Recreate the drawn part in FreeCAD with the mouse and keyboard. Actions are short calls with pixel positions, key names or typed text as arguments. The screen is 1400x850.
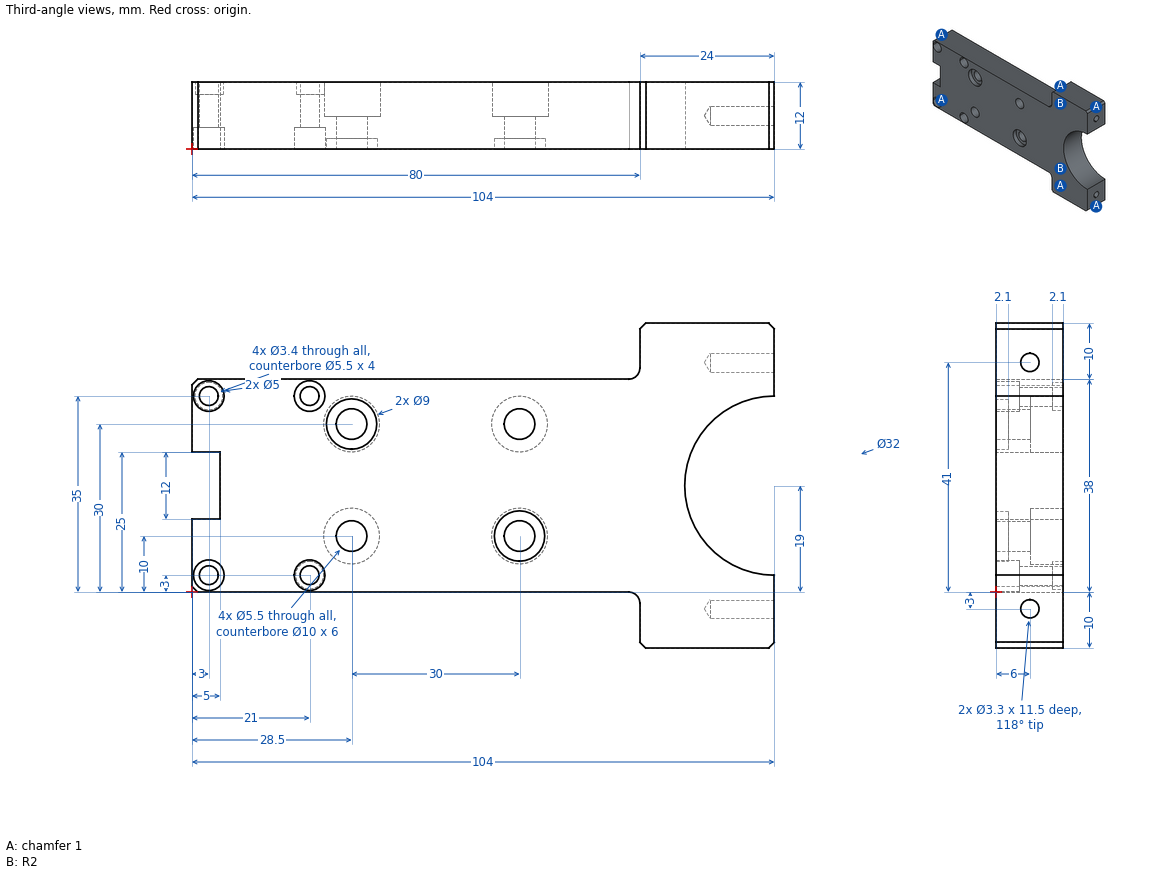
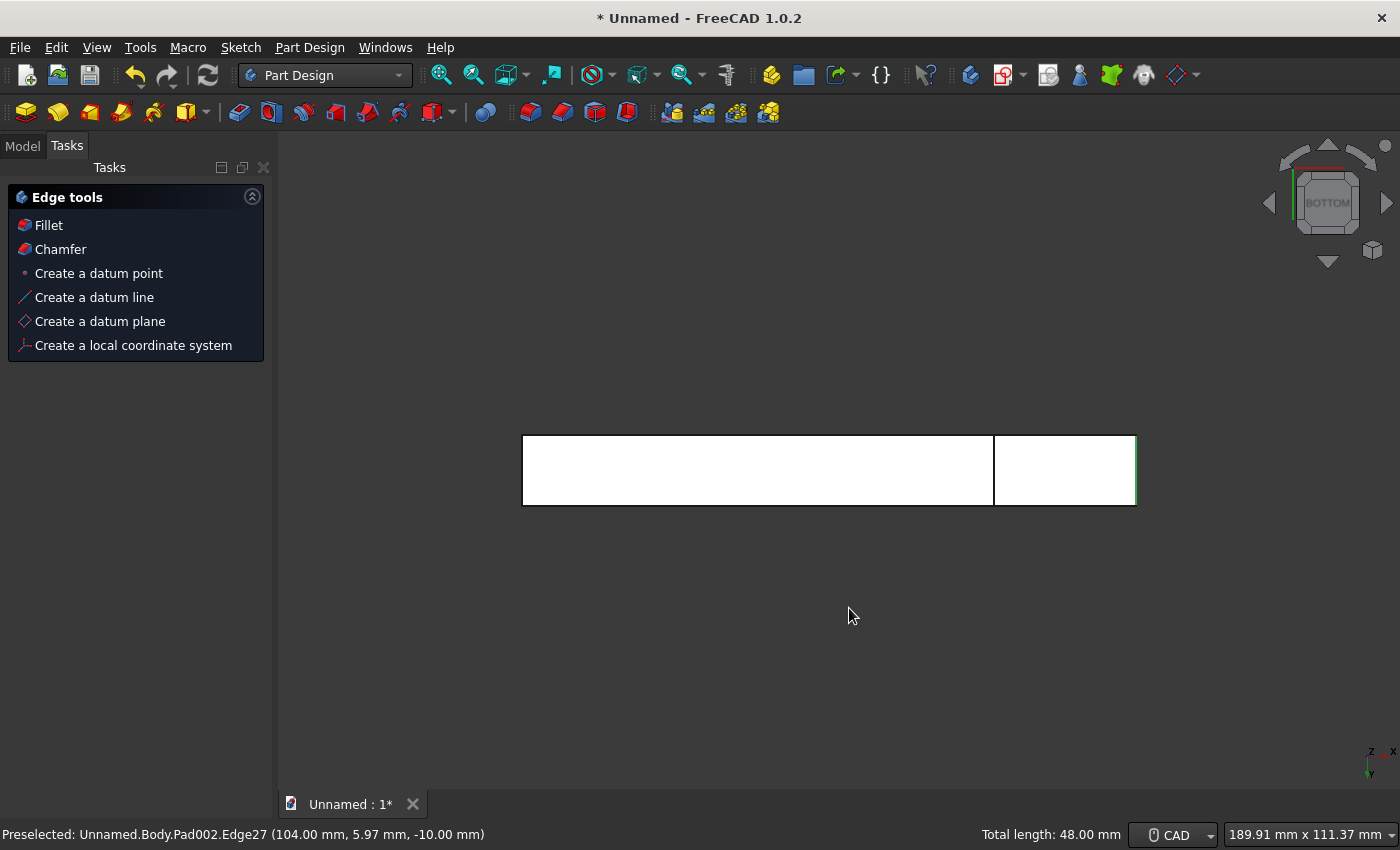
click(522, 469, ctrl)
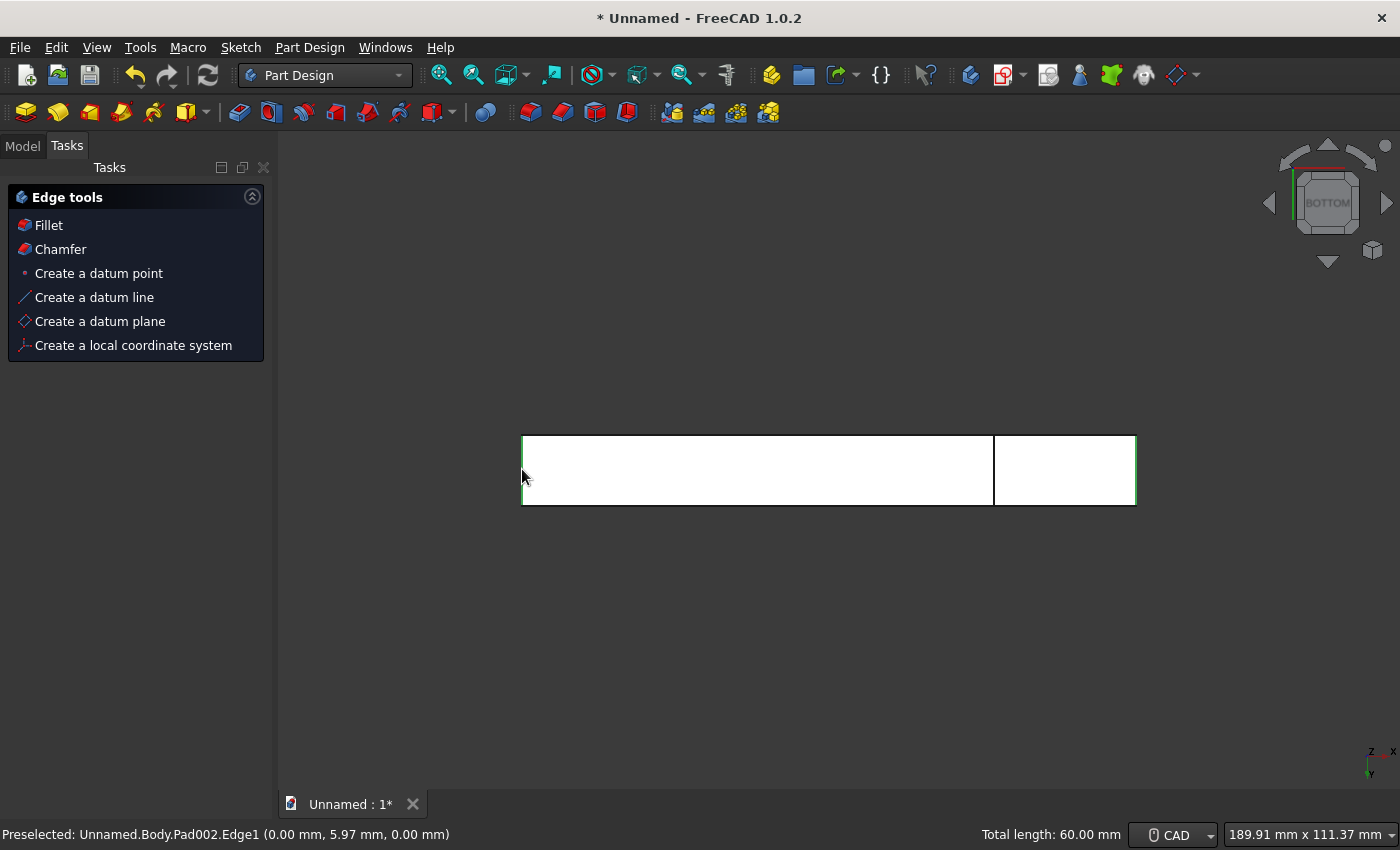
click(994, 469, ctrl)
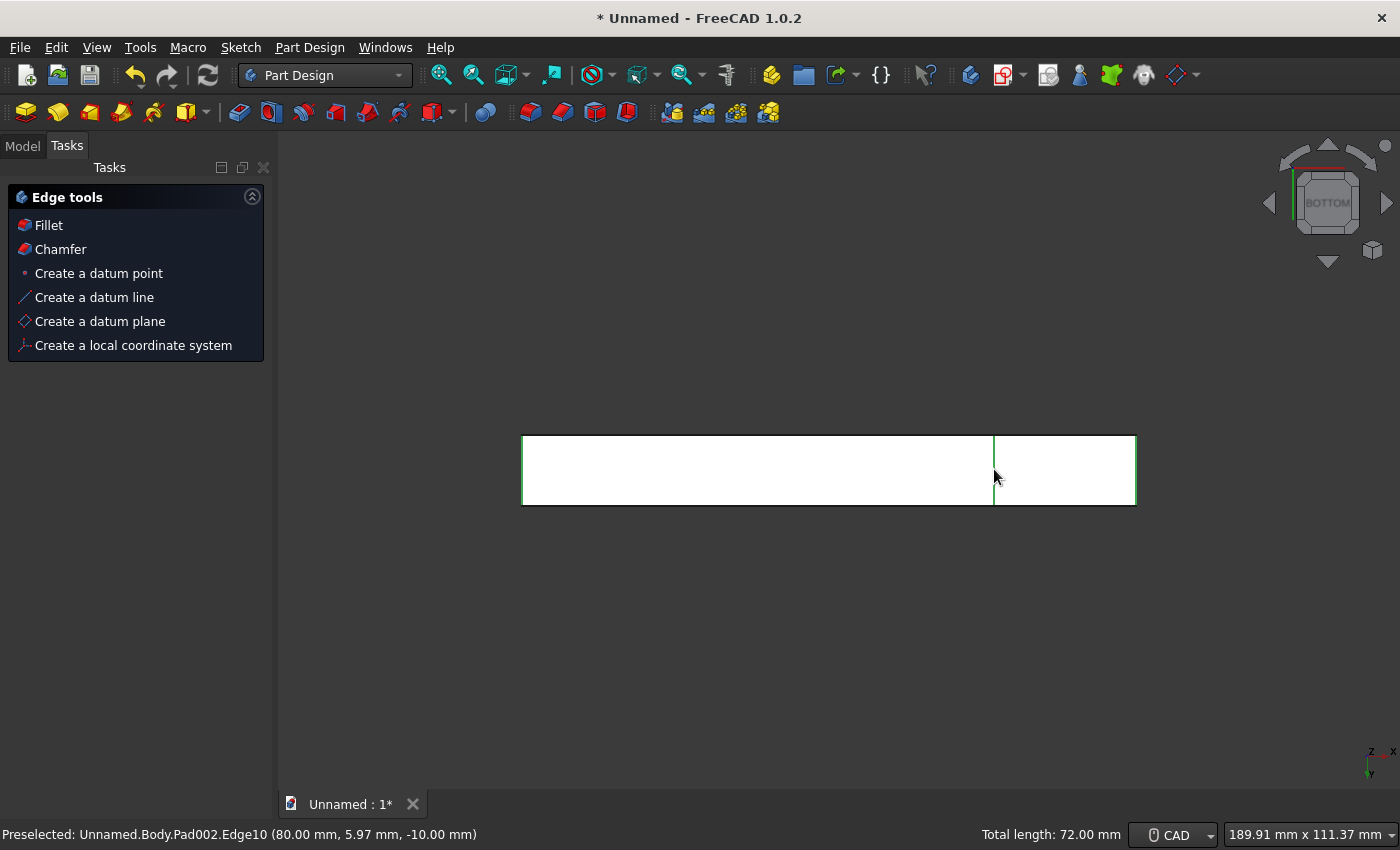
click(564, 112)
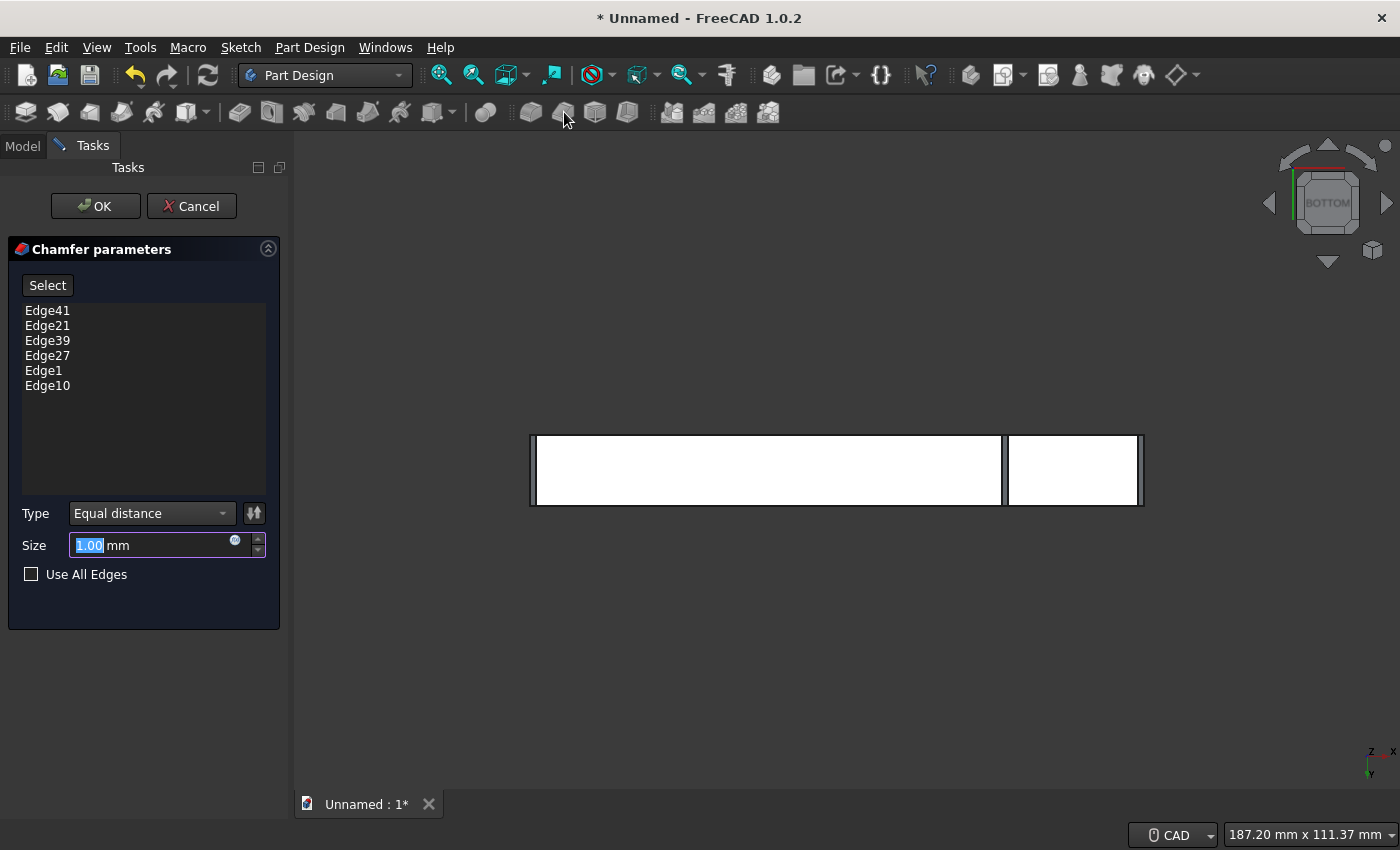
text(1)
key(Tab)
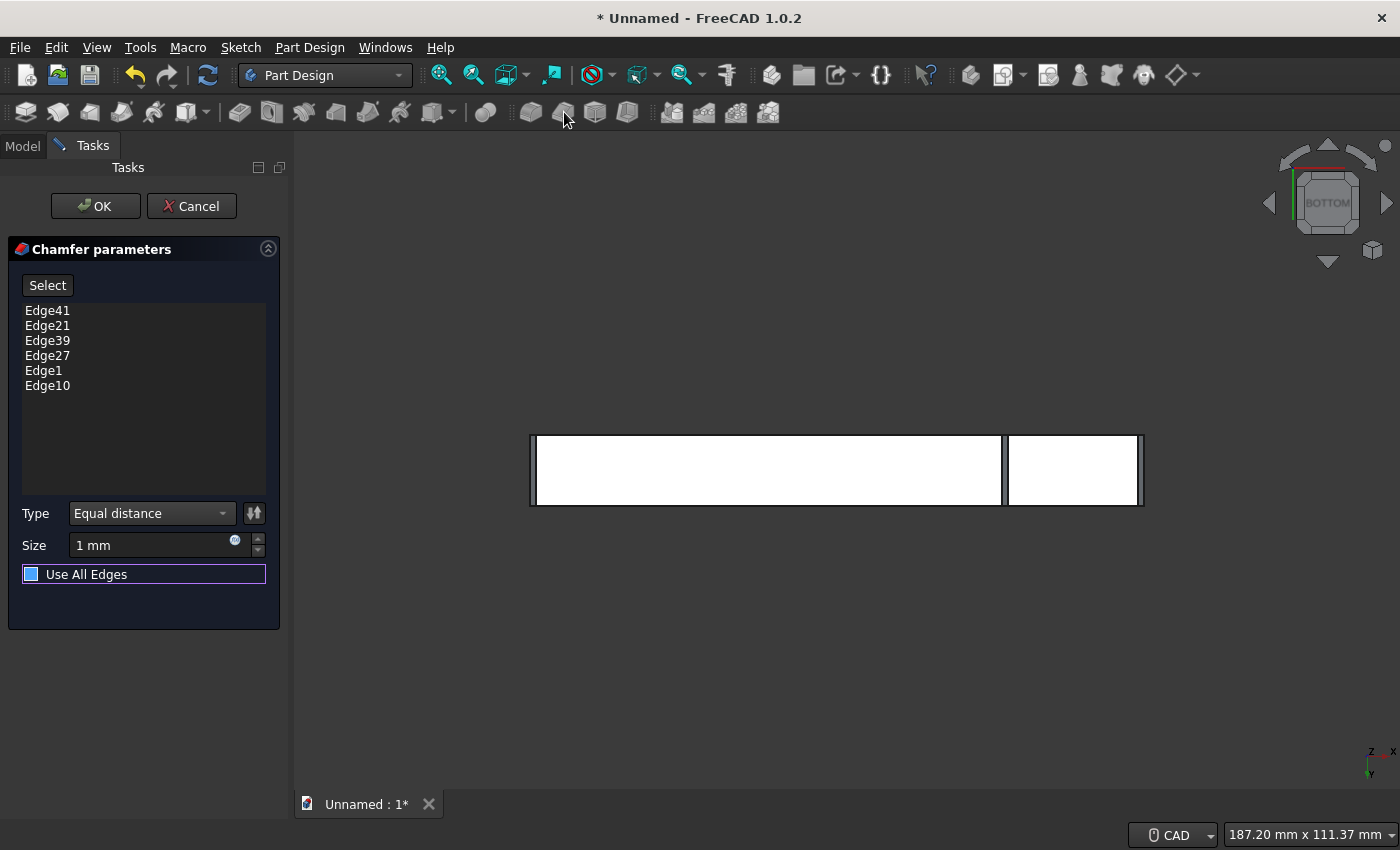
click(96, 206)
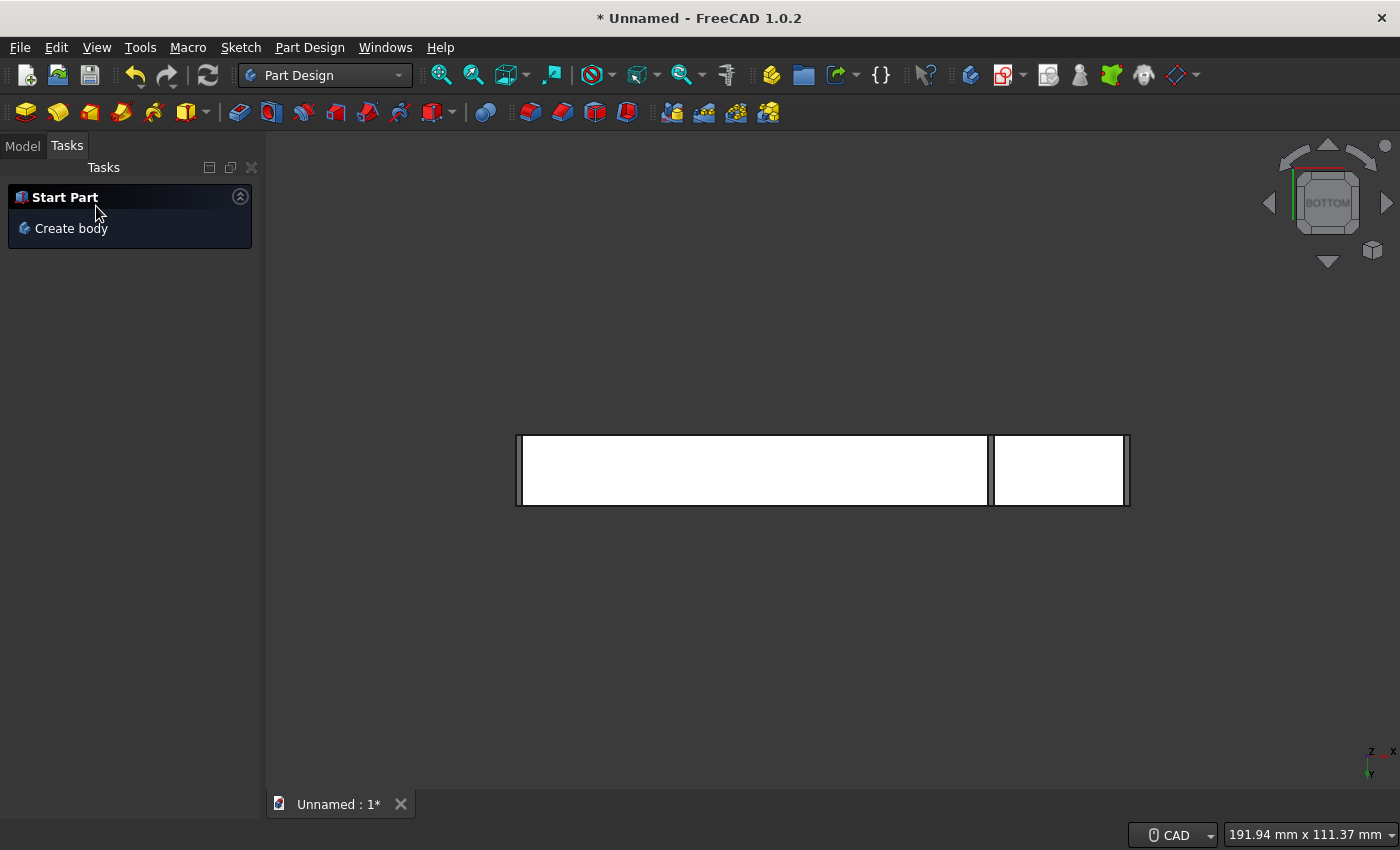
key(0)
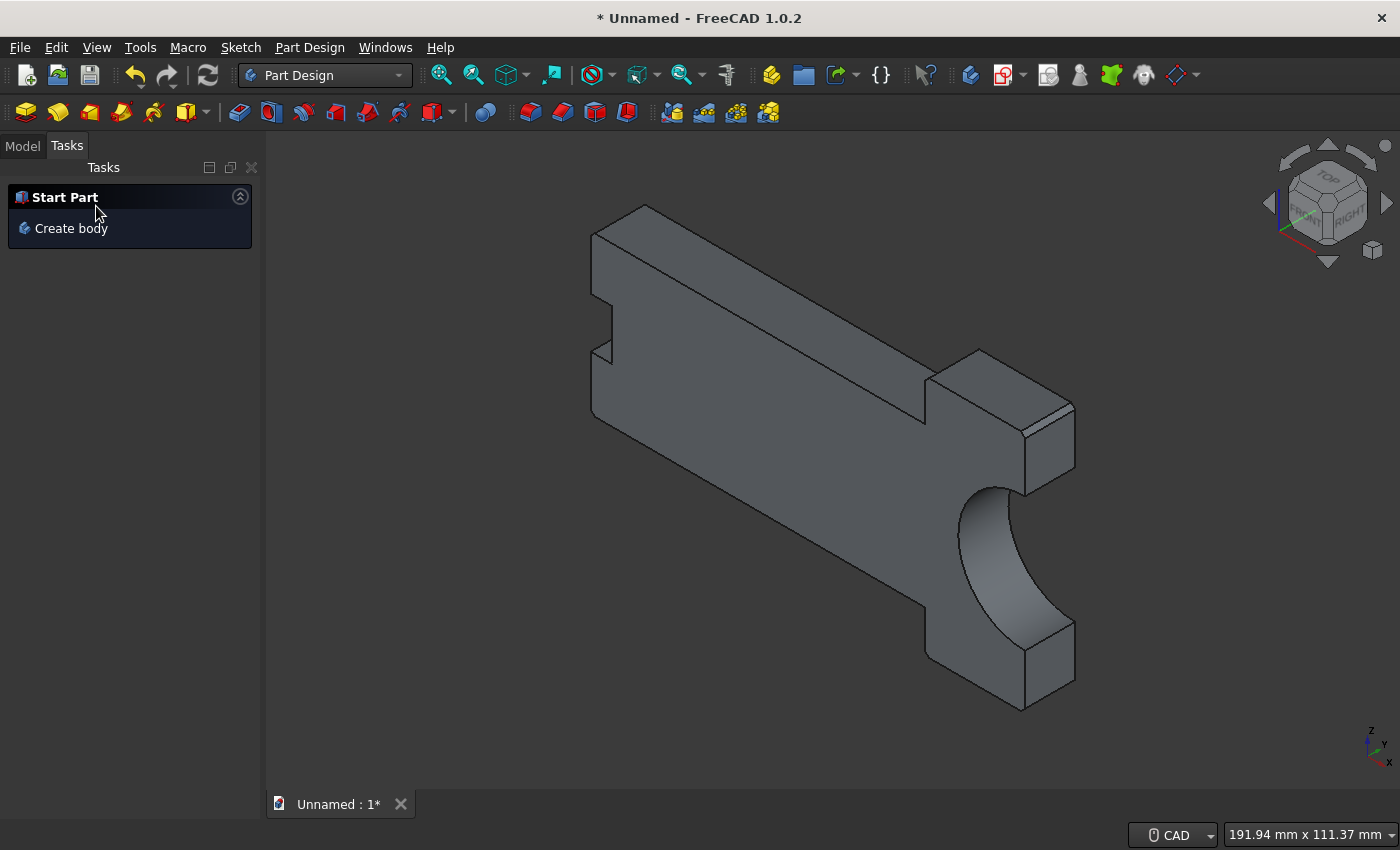
key(2)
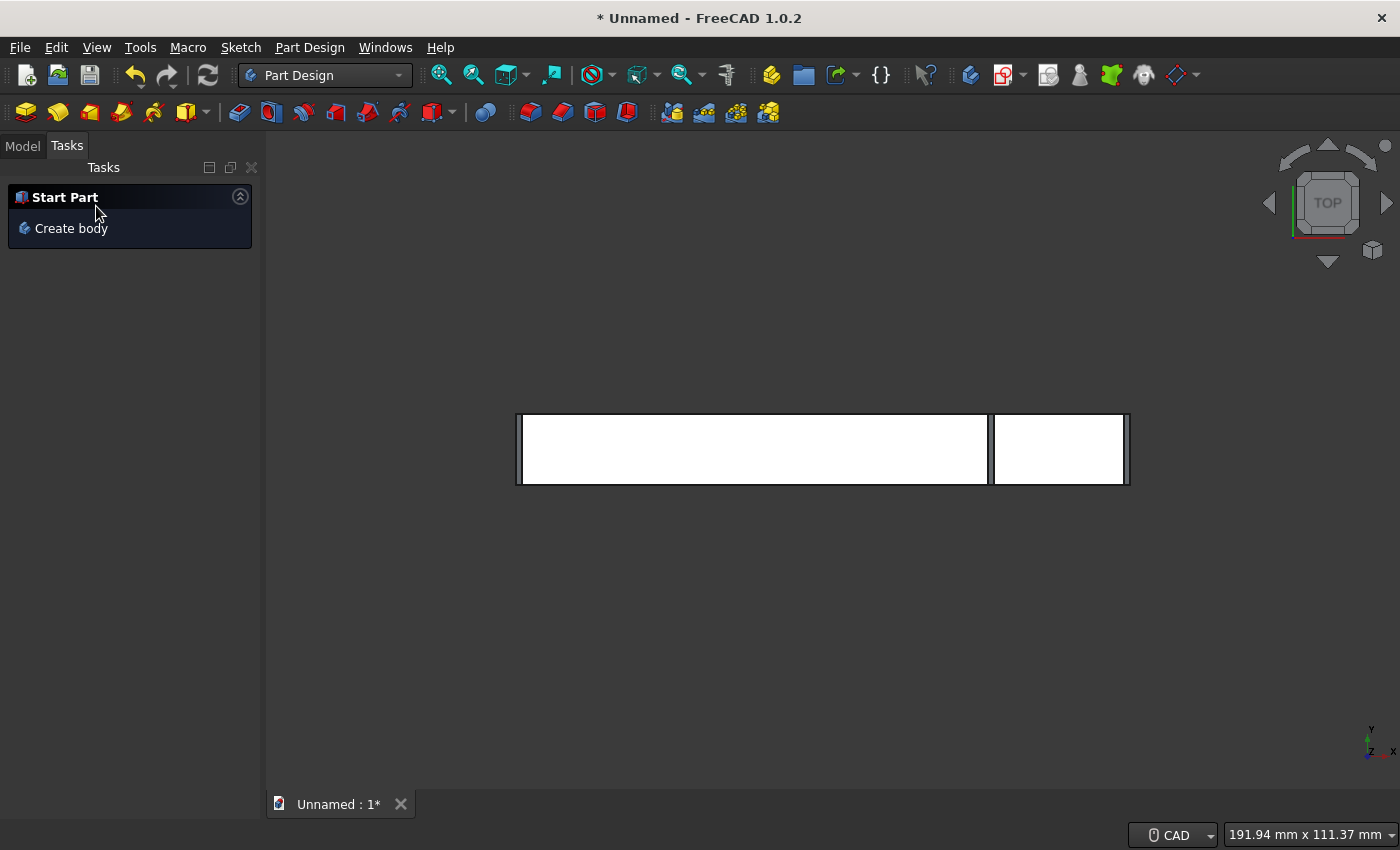
key(1)